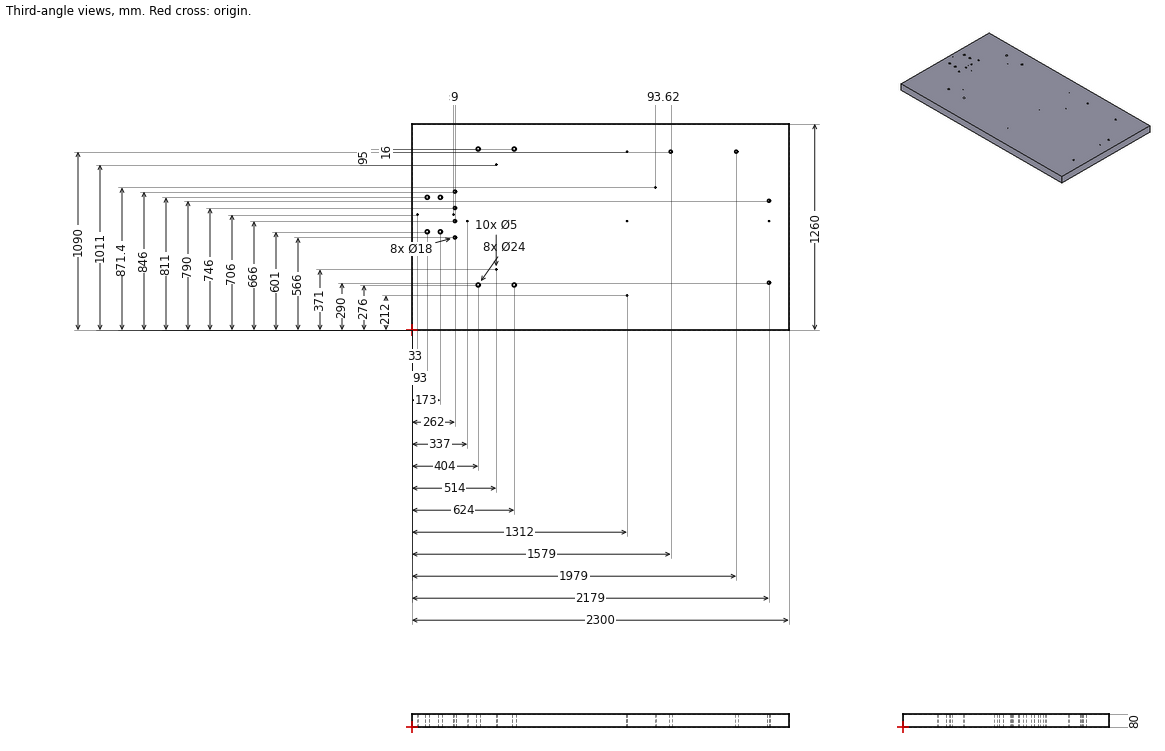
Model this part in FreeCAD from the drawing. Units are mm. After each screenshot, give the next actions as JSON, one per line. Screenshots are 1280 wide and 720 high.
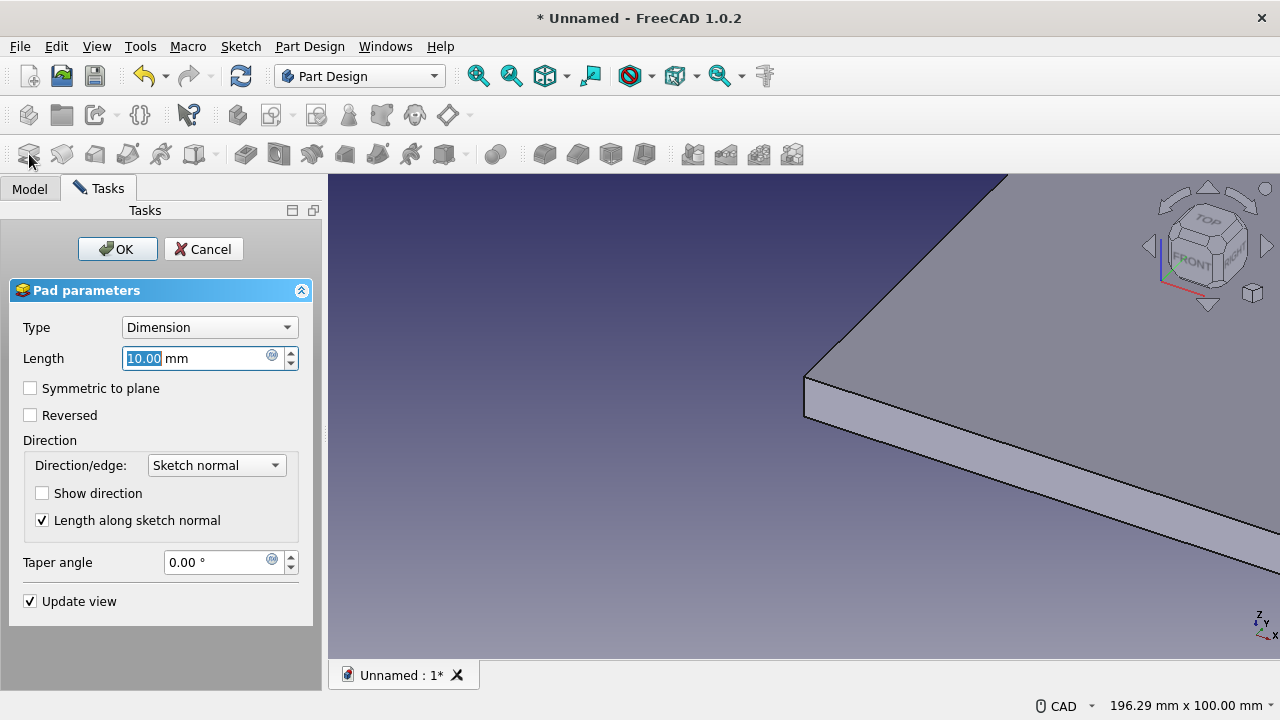
{"action": "type", "text": "80"}
{"action": "key", "text": "Tab"}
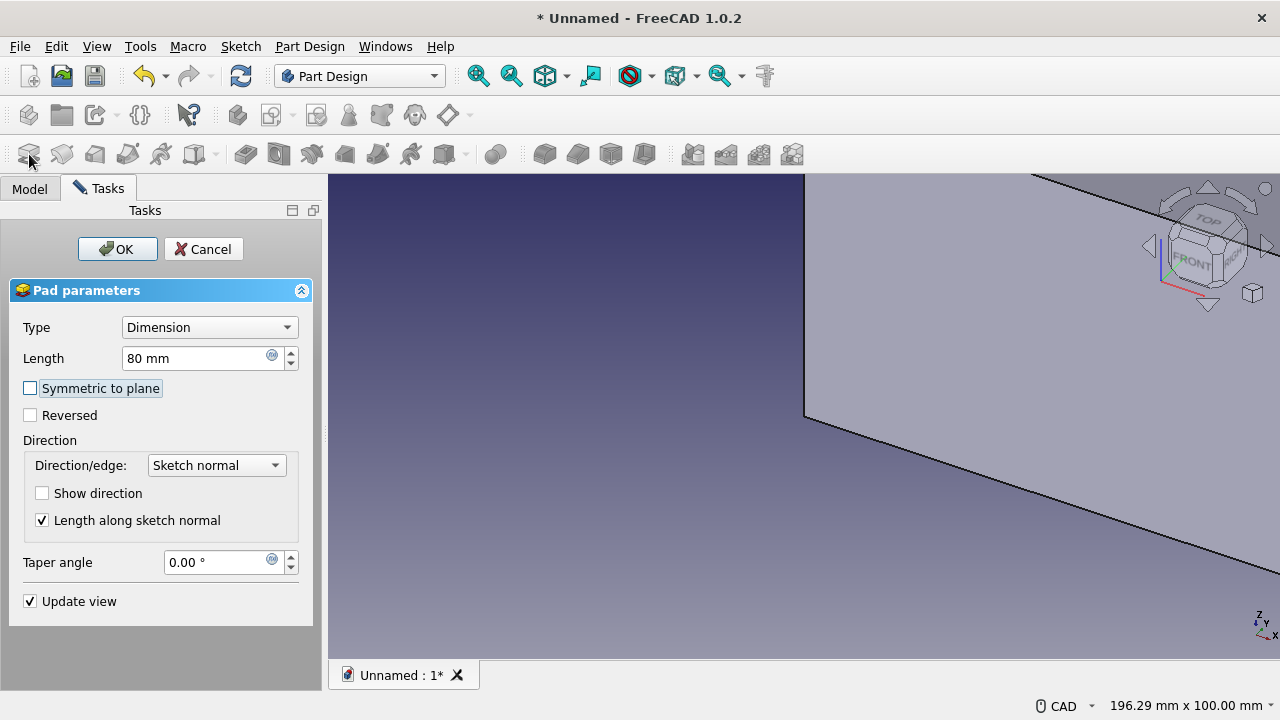
{"action": "left_click", "coordinate": [118, 249]}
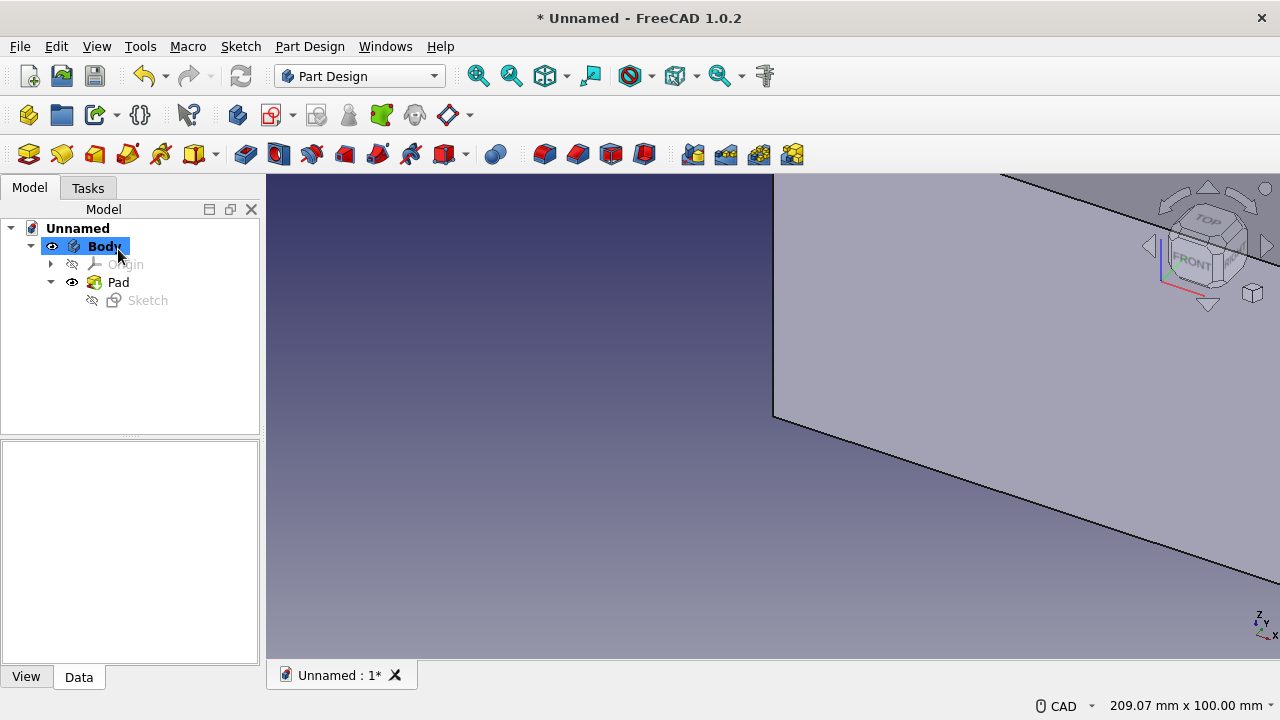
{"action": "key", "text": "0"}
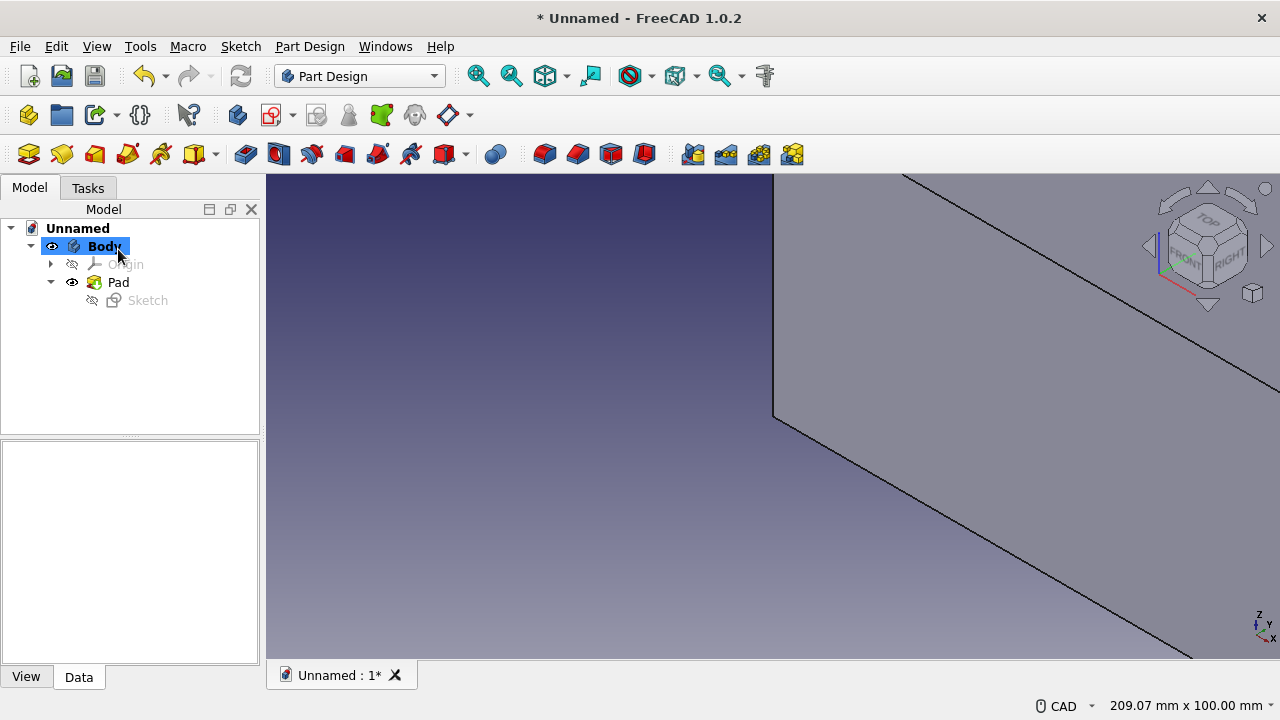
{"action": "left_click", "coordinate": [479, 76]}